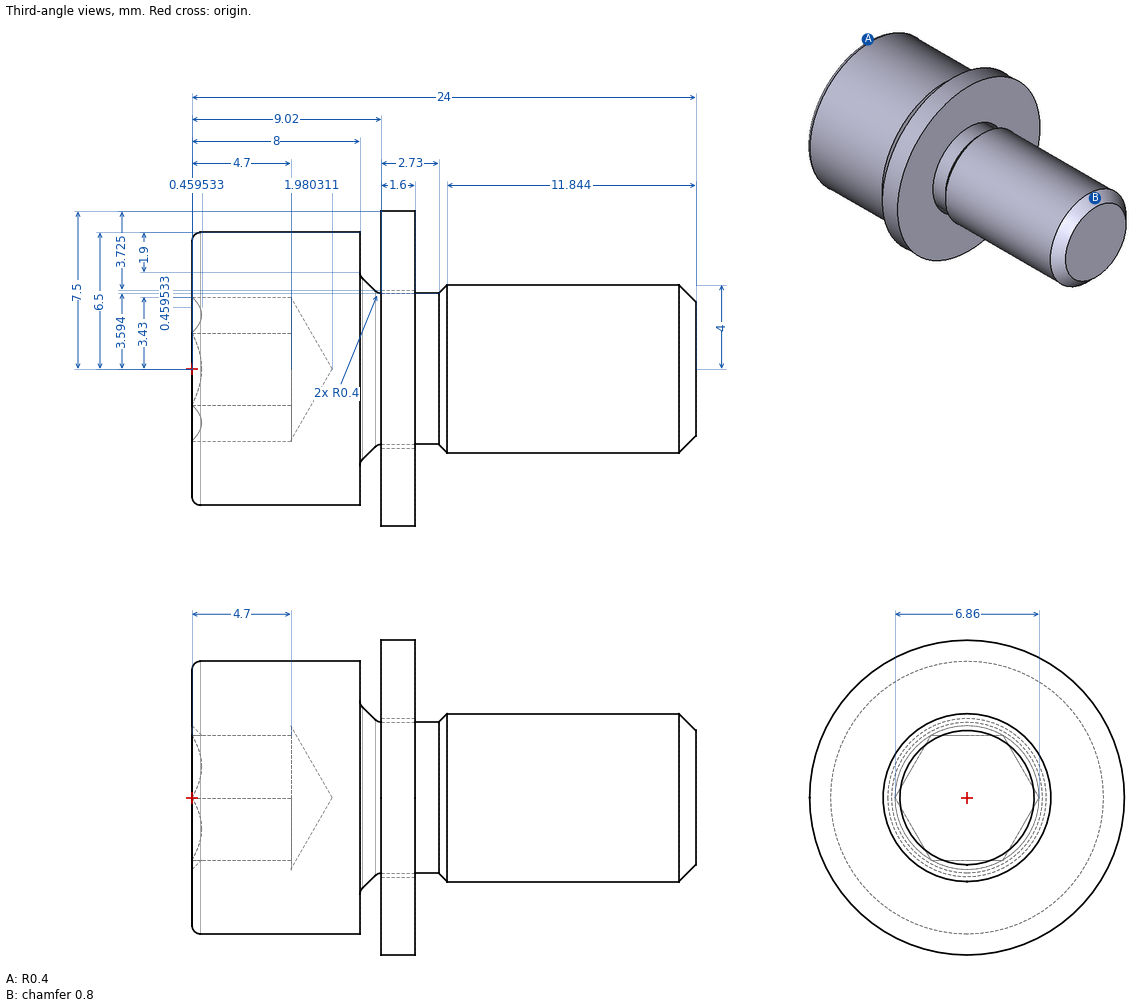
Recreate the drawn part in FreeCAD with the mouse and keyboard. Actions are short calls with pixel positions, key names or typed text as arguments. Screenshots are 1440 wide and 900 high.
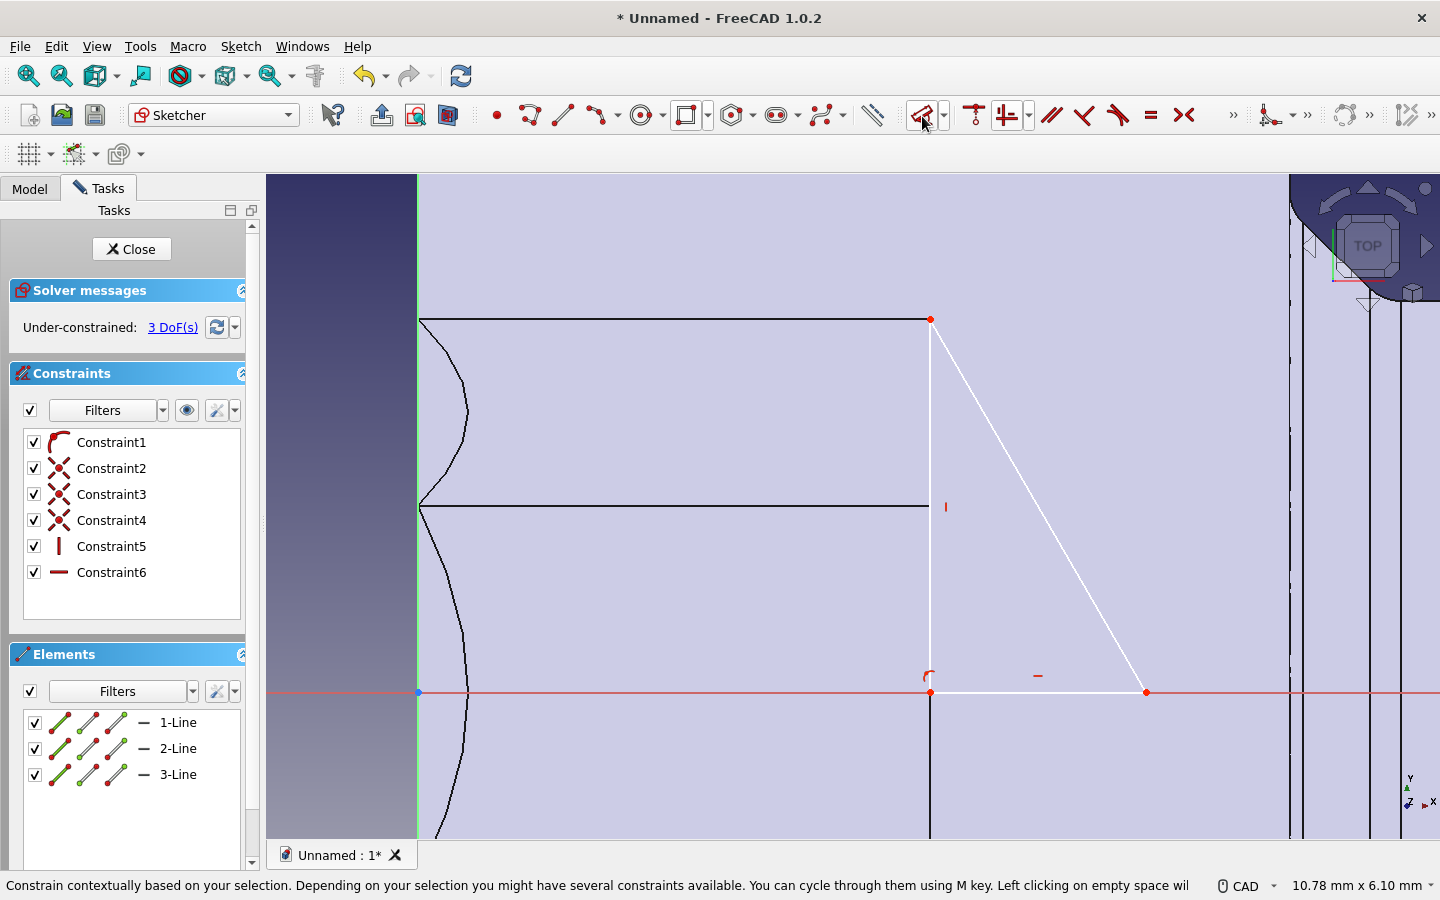
click(930, 432)
click(964, 506)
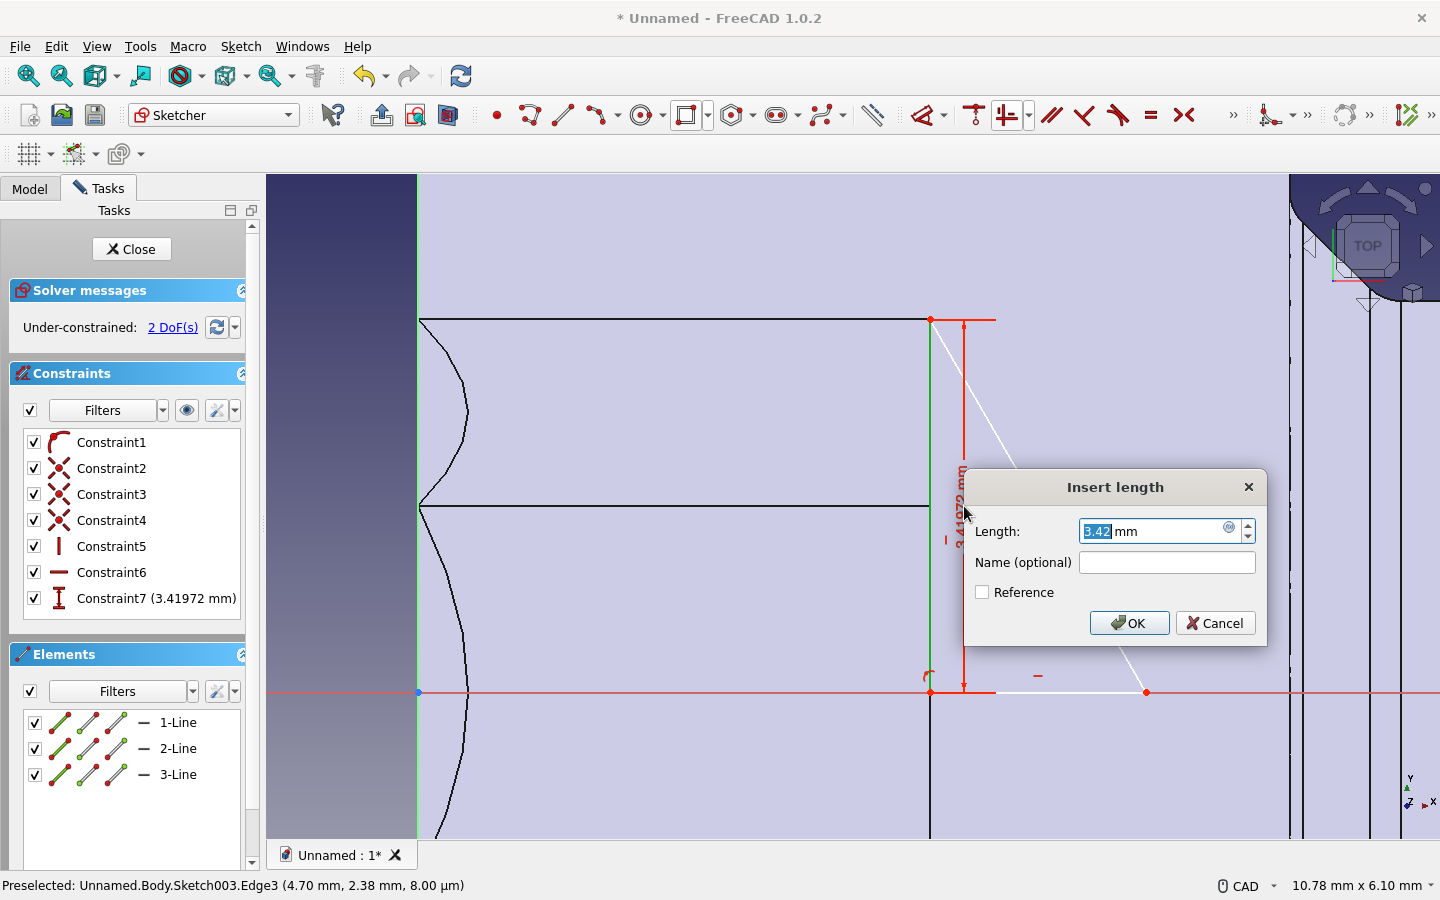
text(3.43)
key(Return)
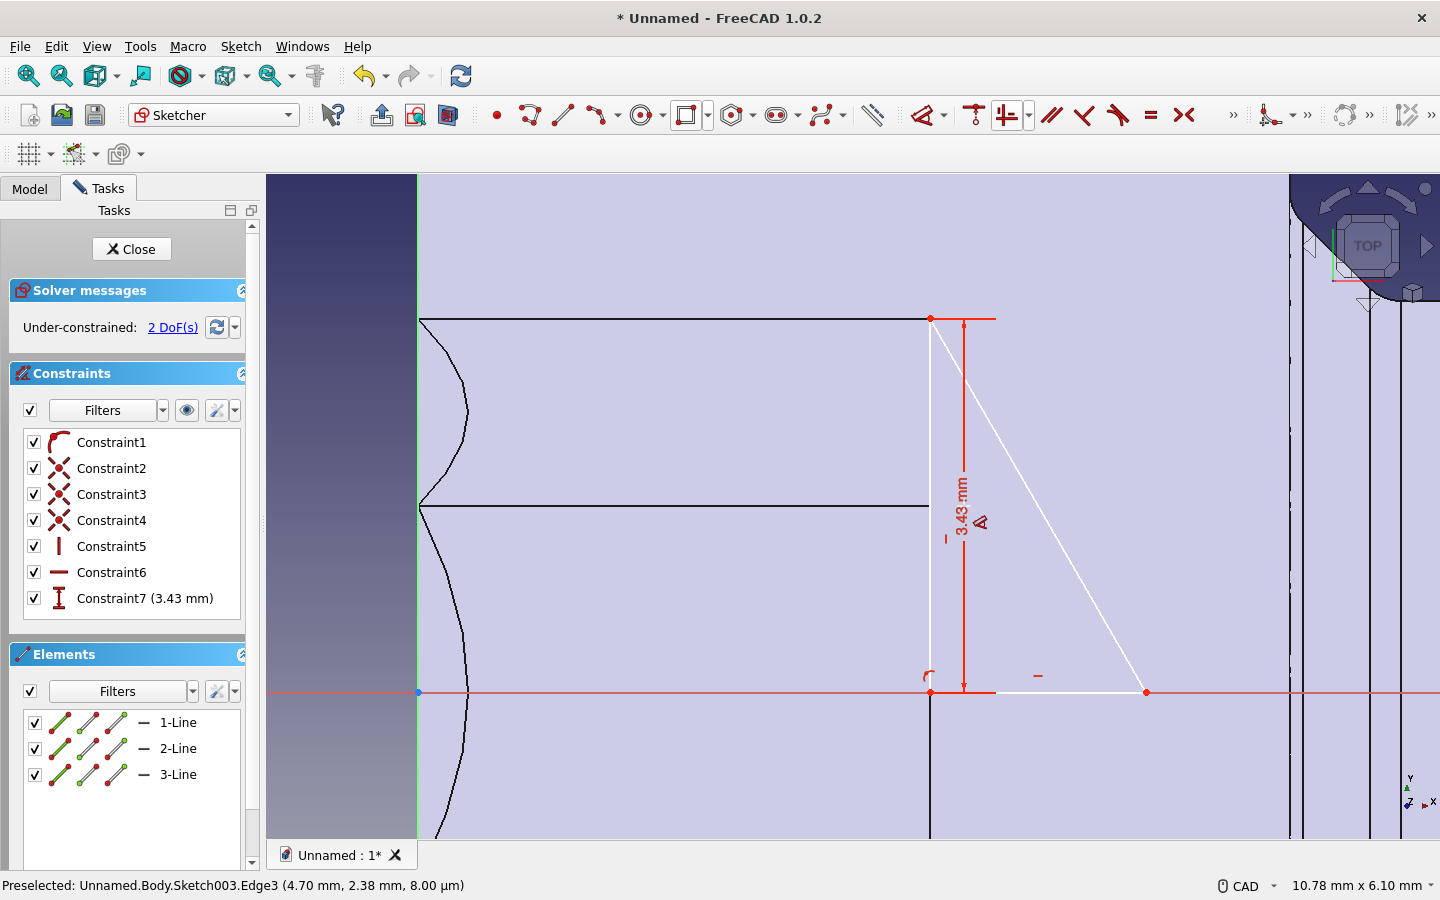
click(930, 693)
click(674, 727)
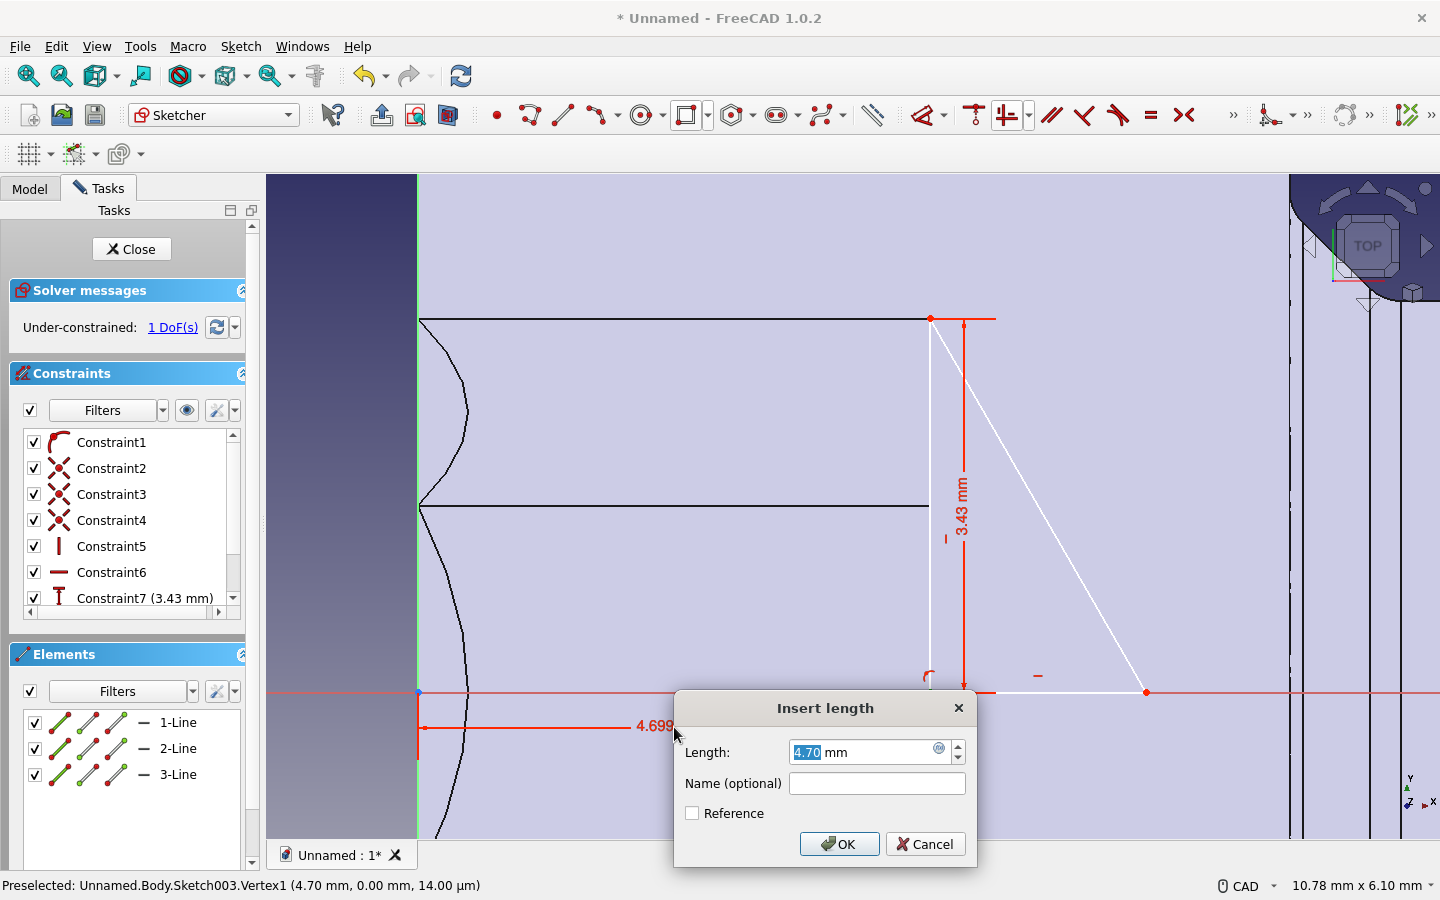
text(4.7)
key(Return)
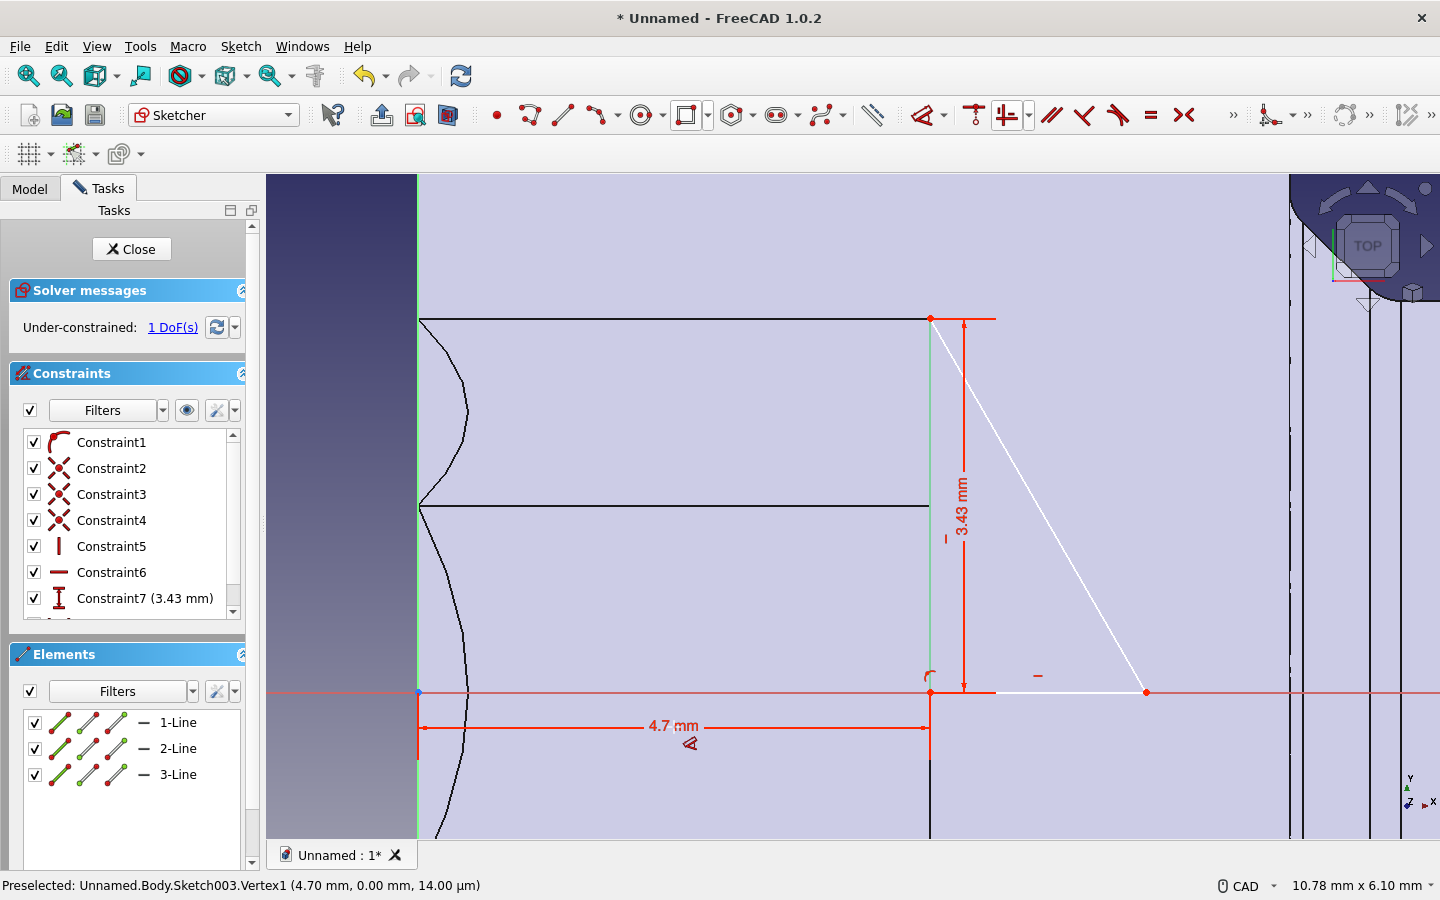
click(995, 693)
click(1038, 727)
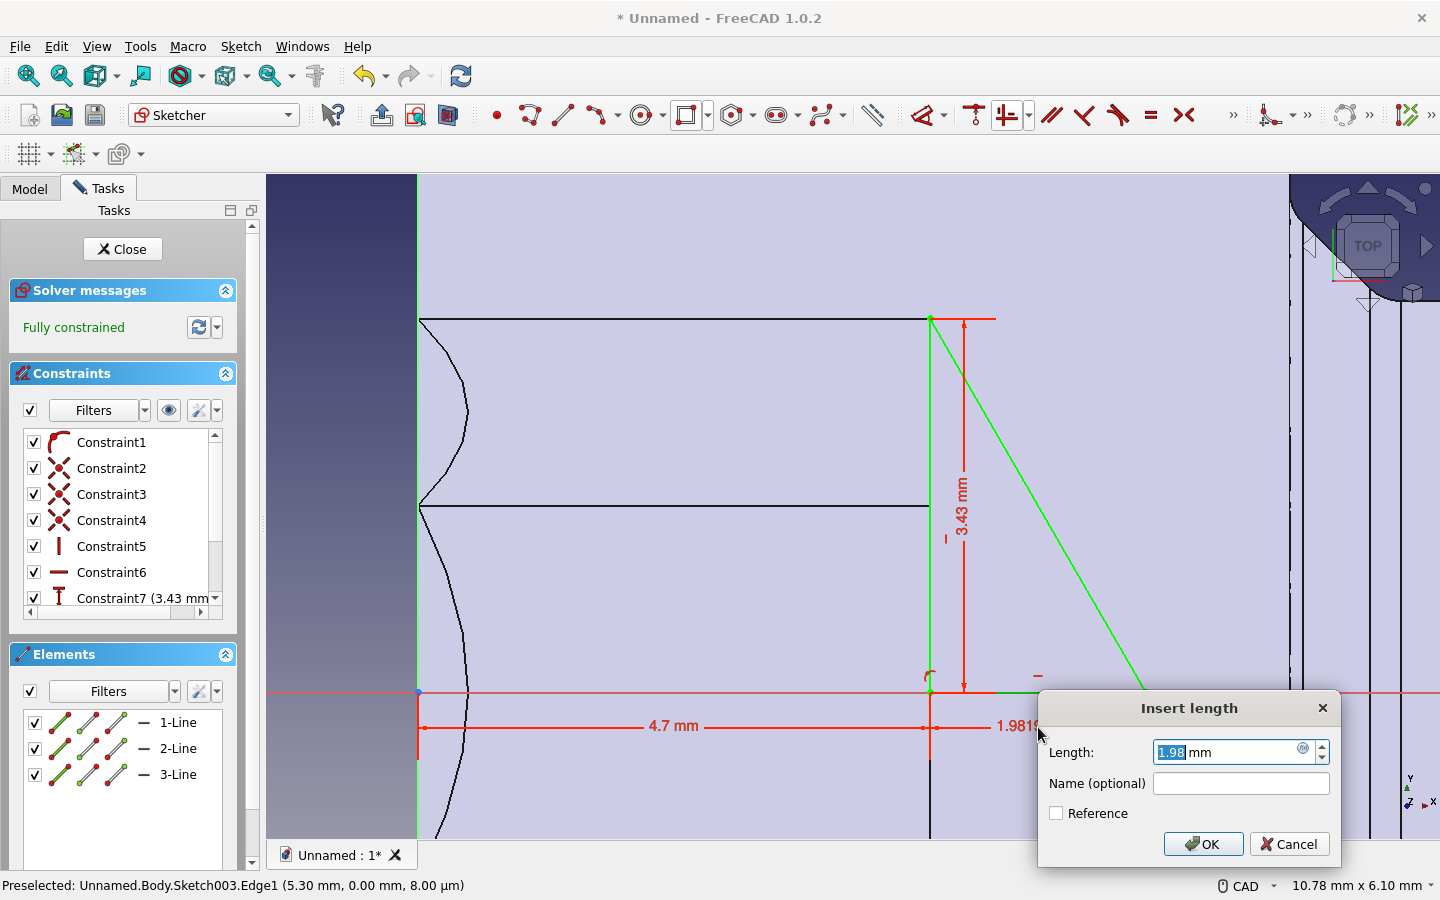
text(1.980311)
key(Return)
key(Escape)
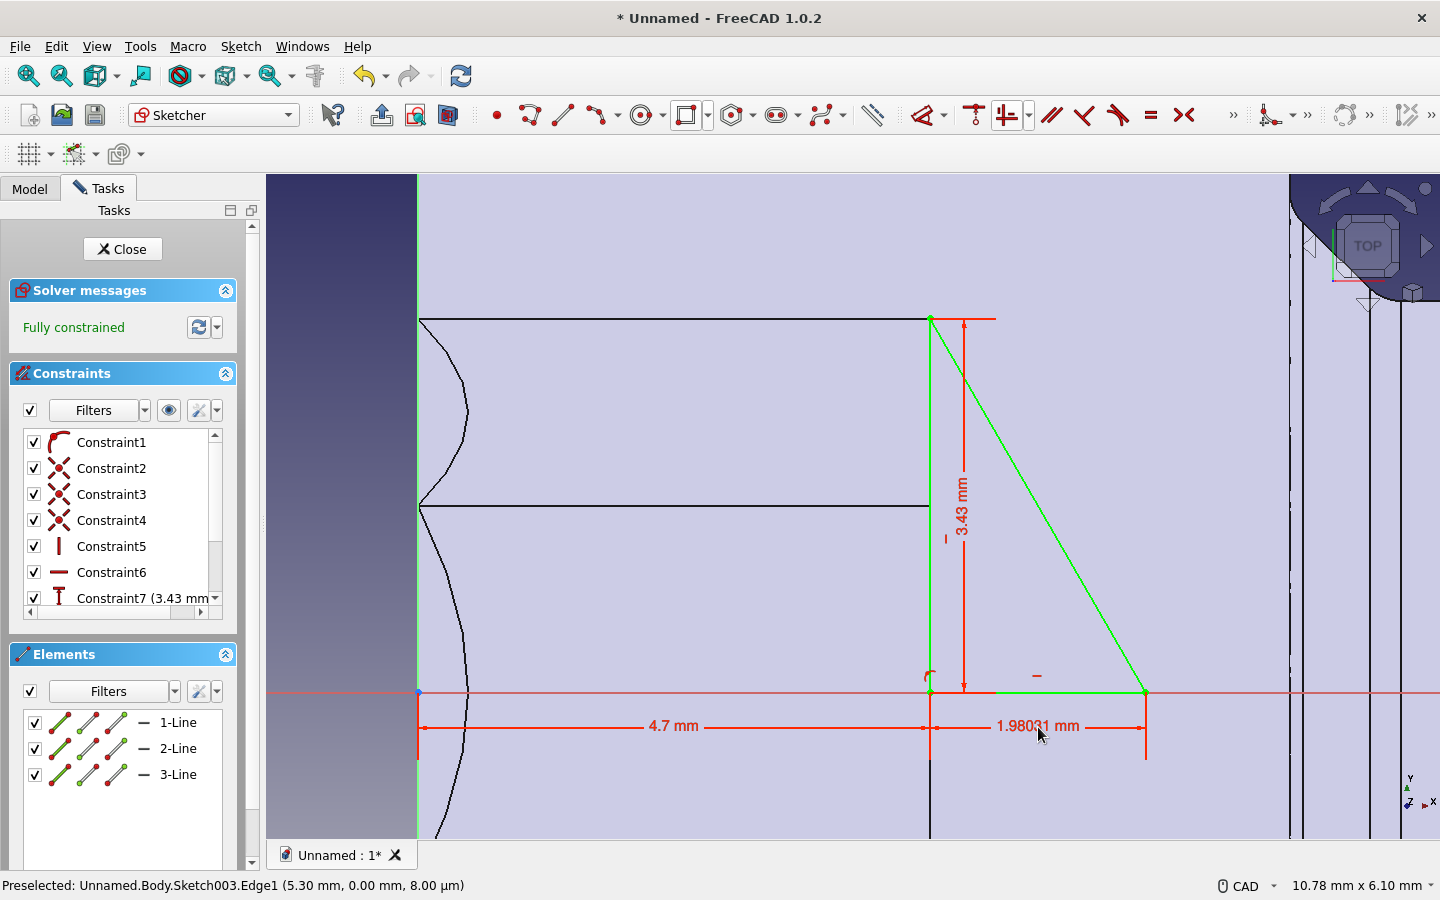
click(123, 249)